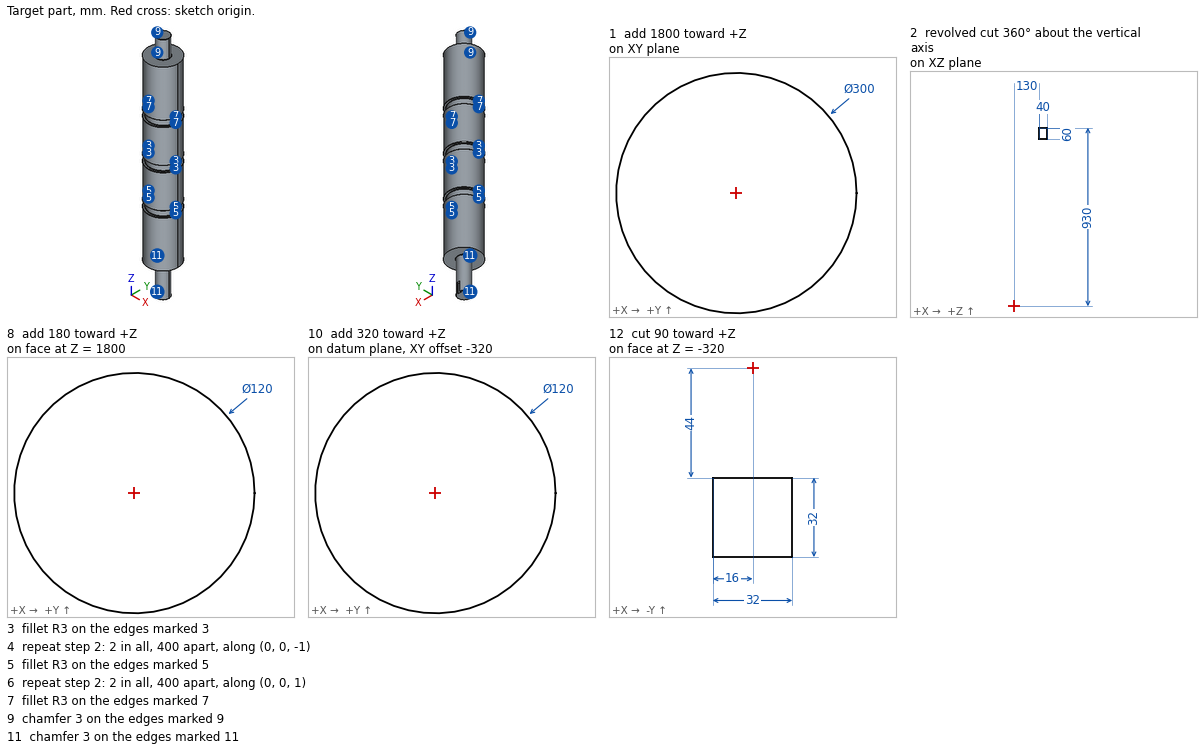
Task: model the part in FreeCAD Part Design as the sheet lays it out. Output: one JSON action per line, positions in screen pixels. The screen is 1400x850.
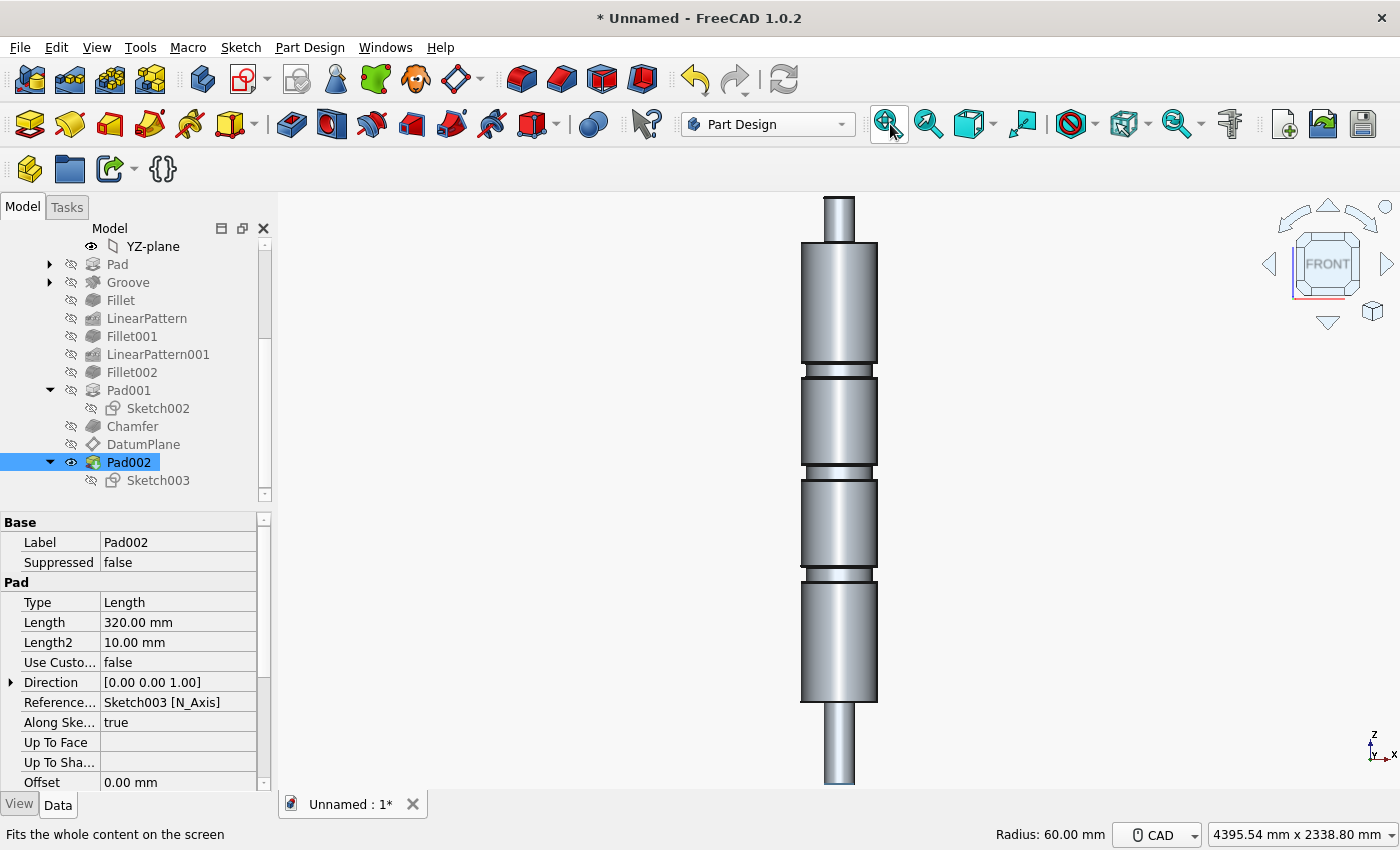
{"action": "key", "text": "3"}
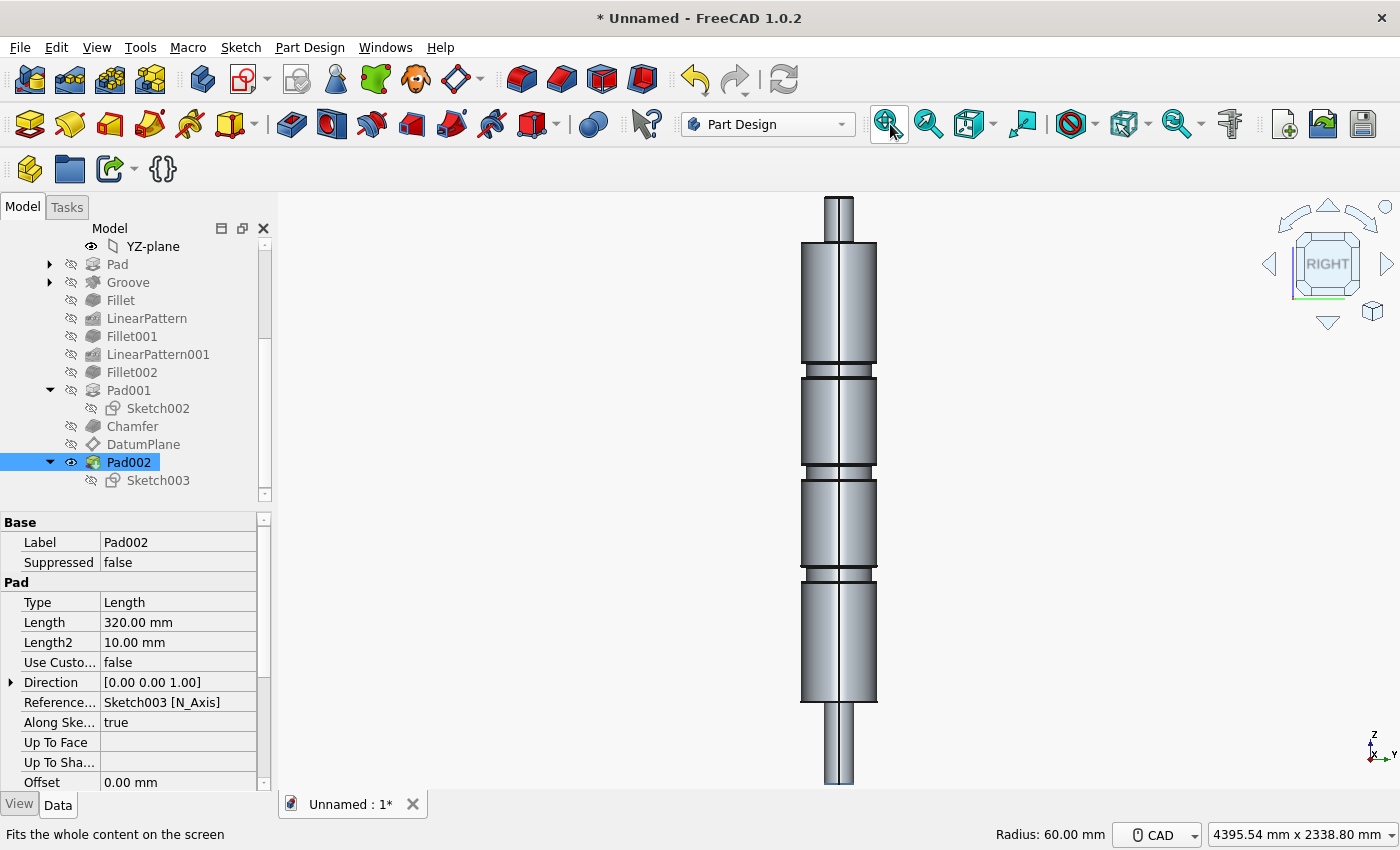
{"action": "key", "text": "5"}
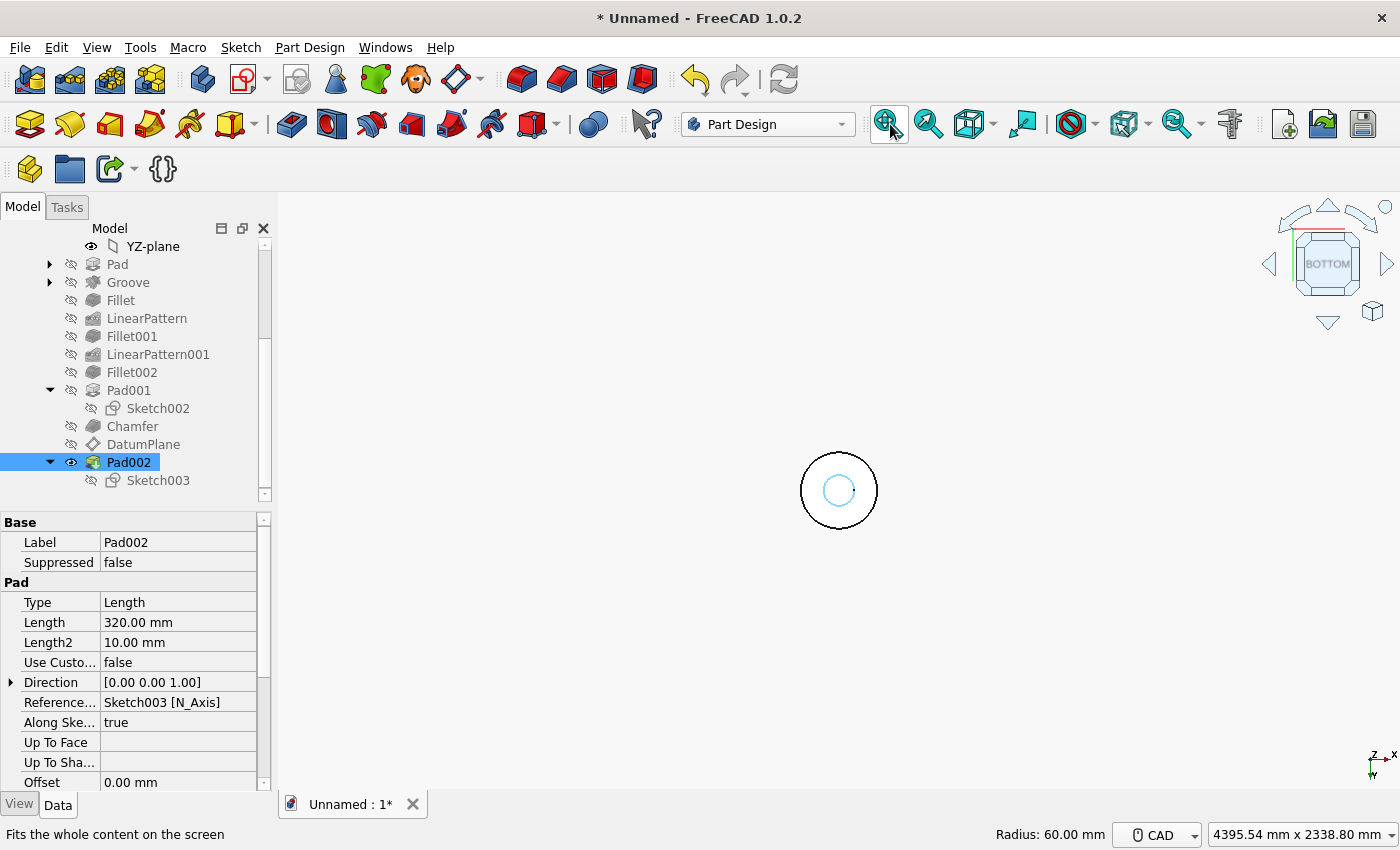
{"action": "left_click", "coordinate": [890, 124]}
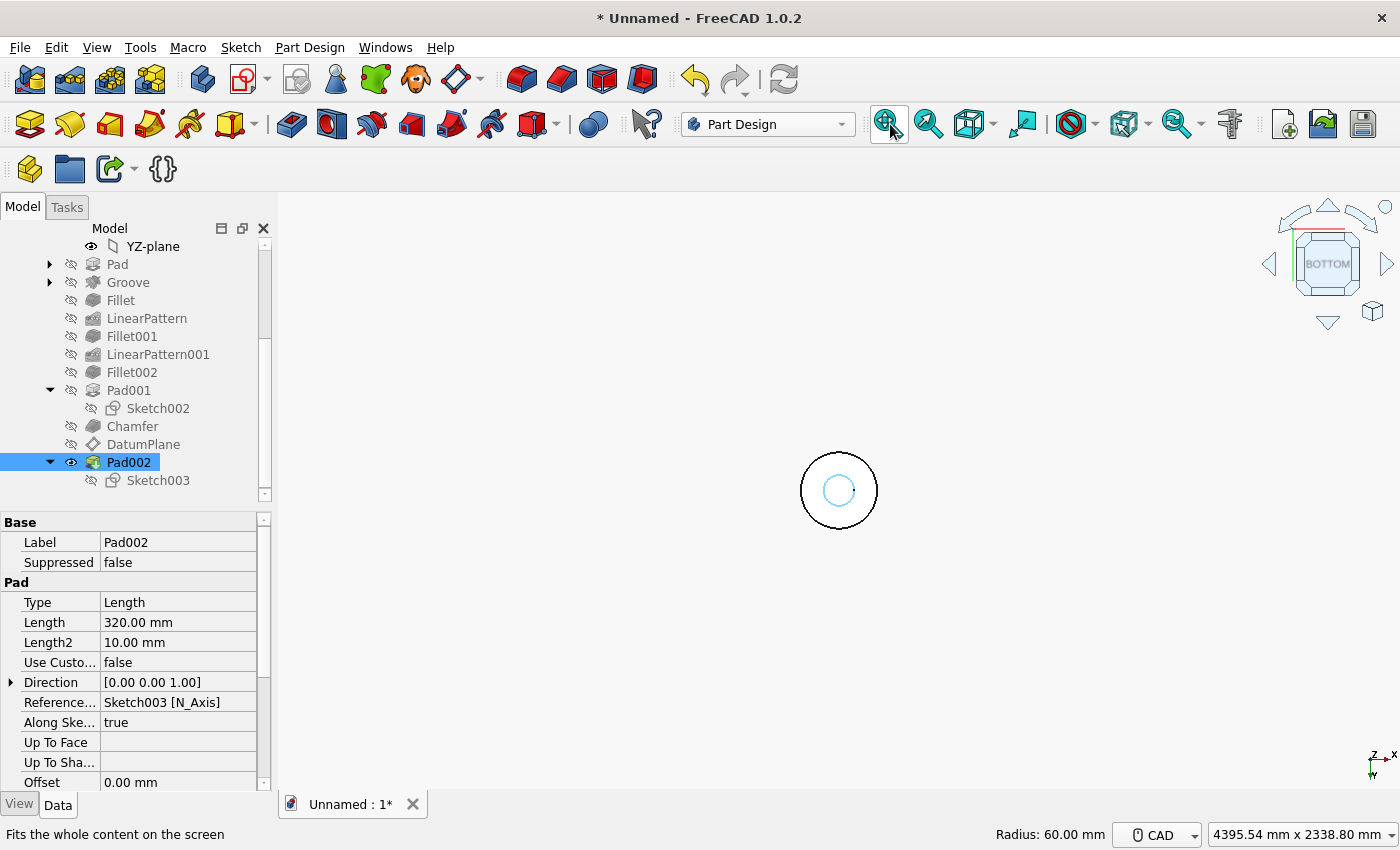
{"action": "key", "text": "4"}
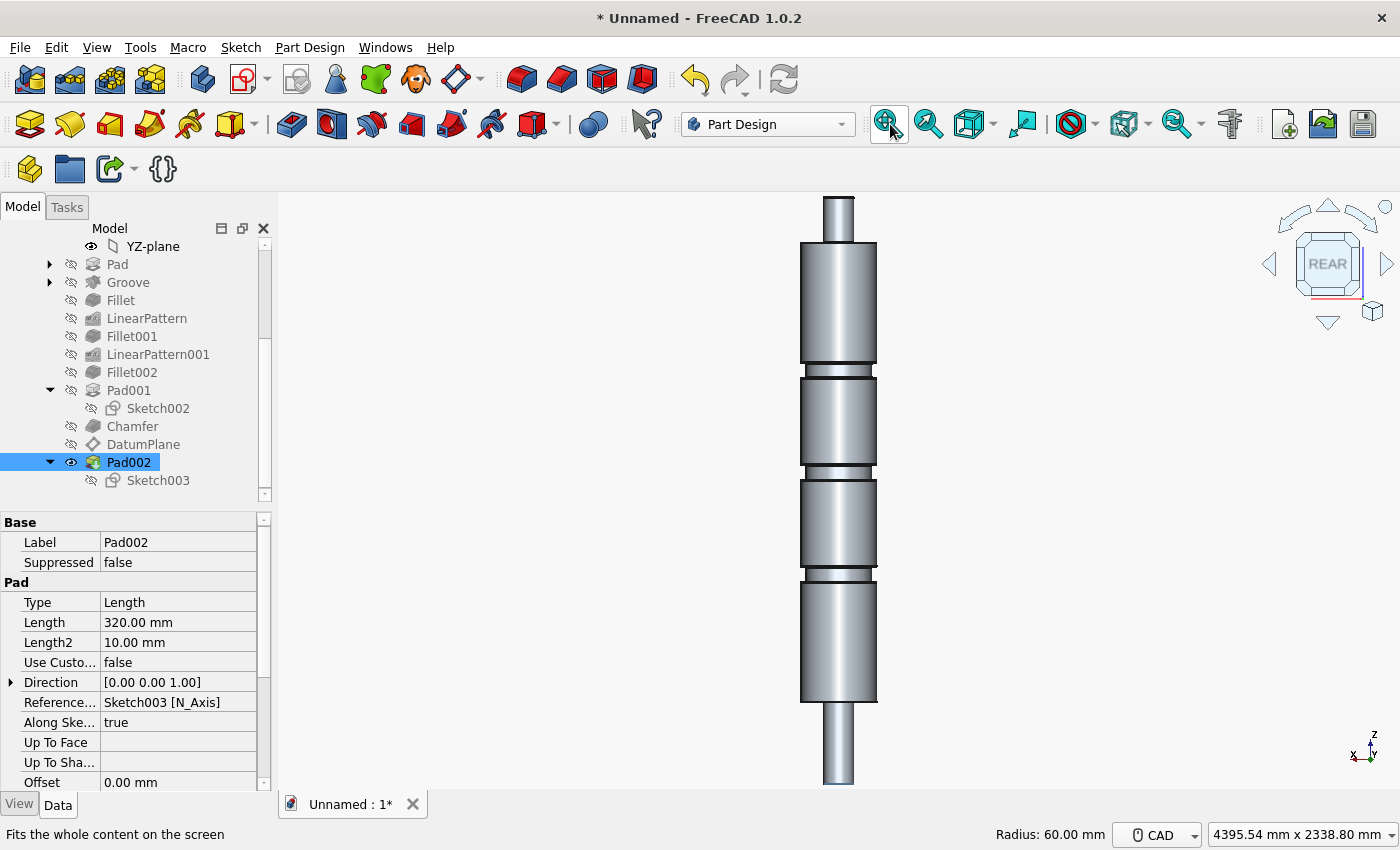
{"action": "key", "text": "6"}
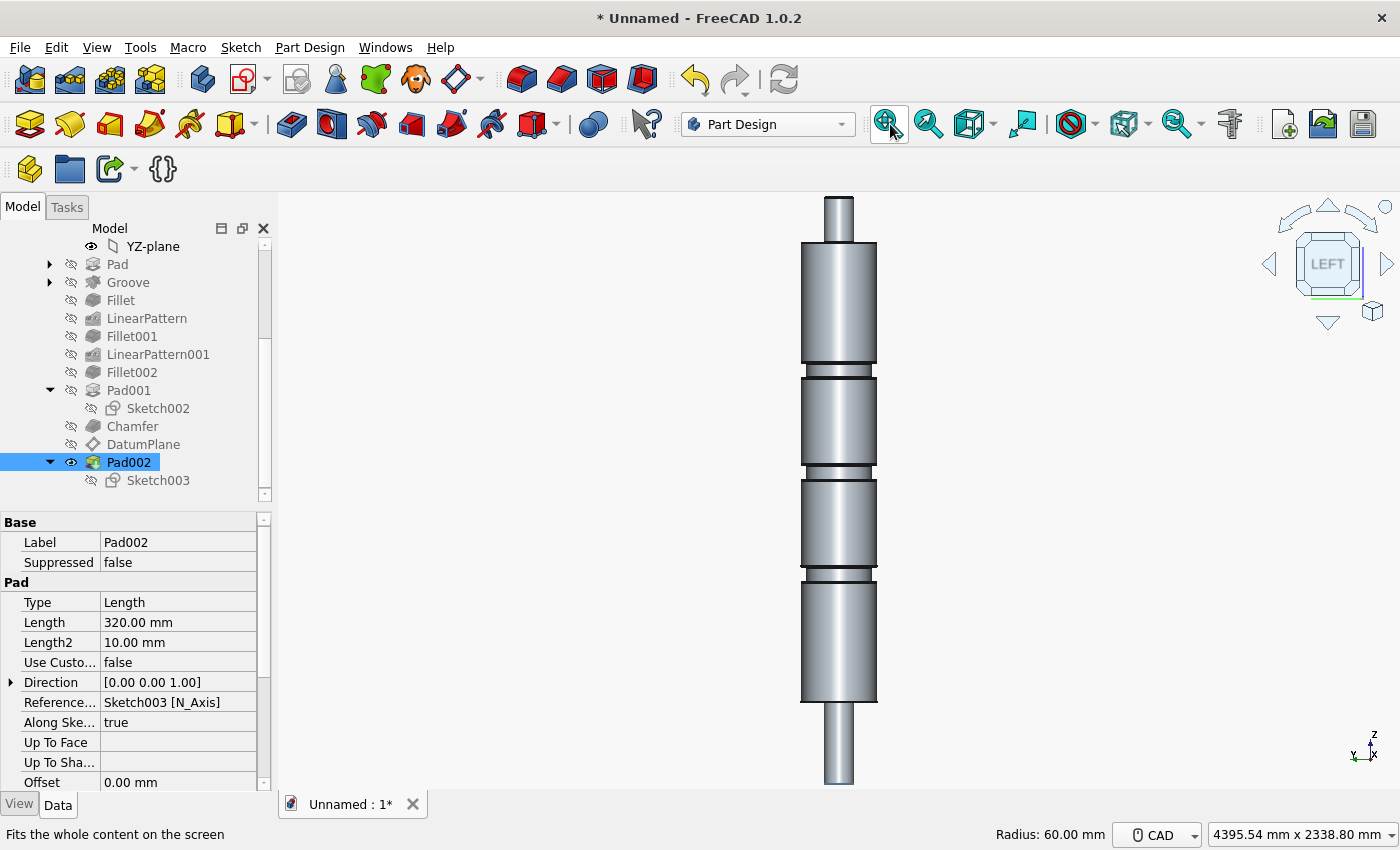
{"action": "key", "text": "v 3"}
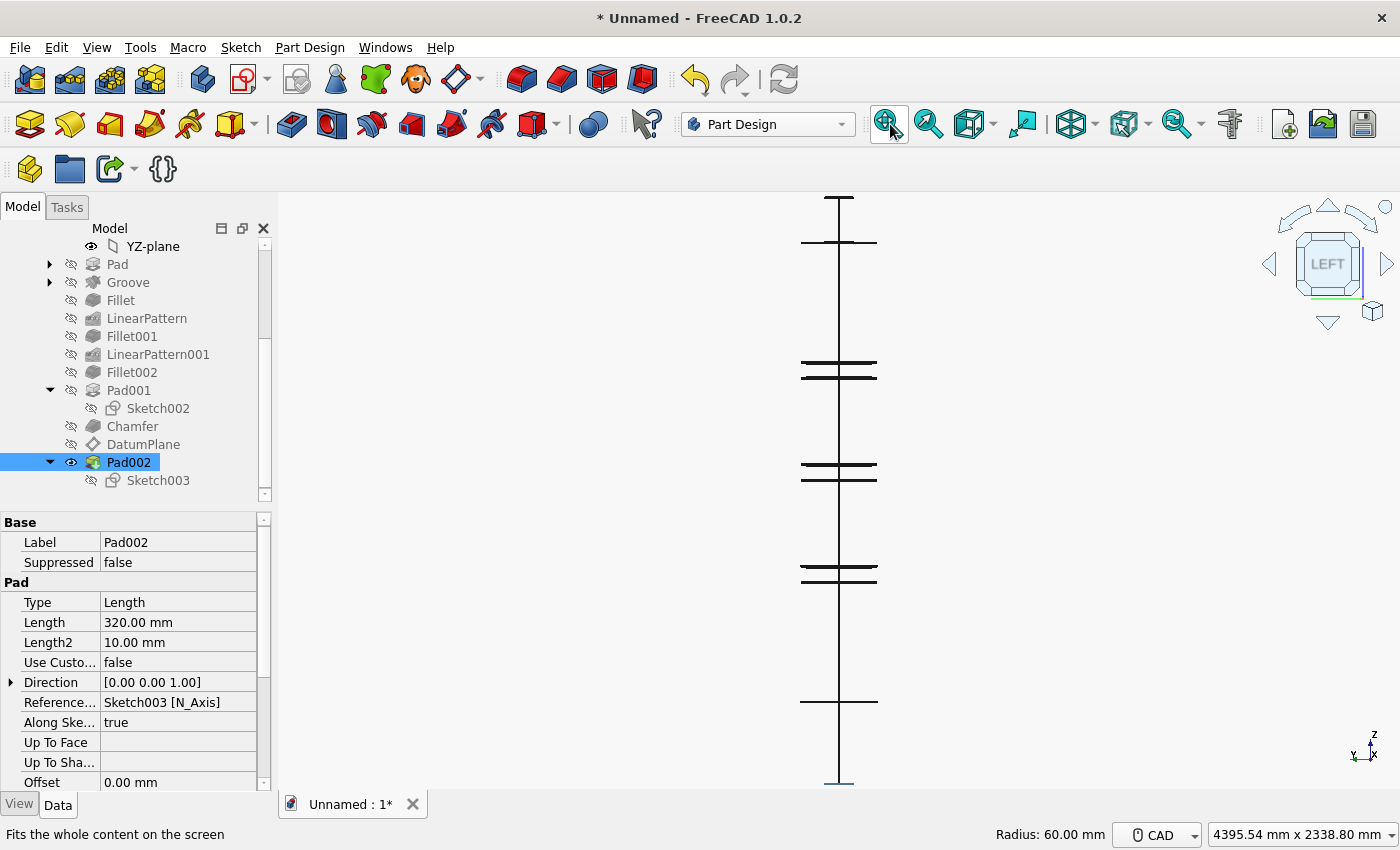
{"action": "key", "text": "0"}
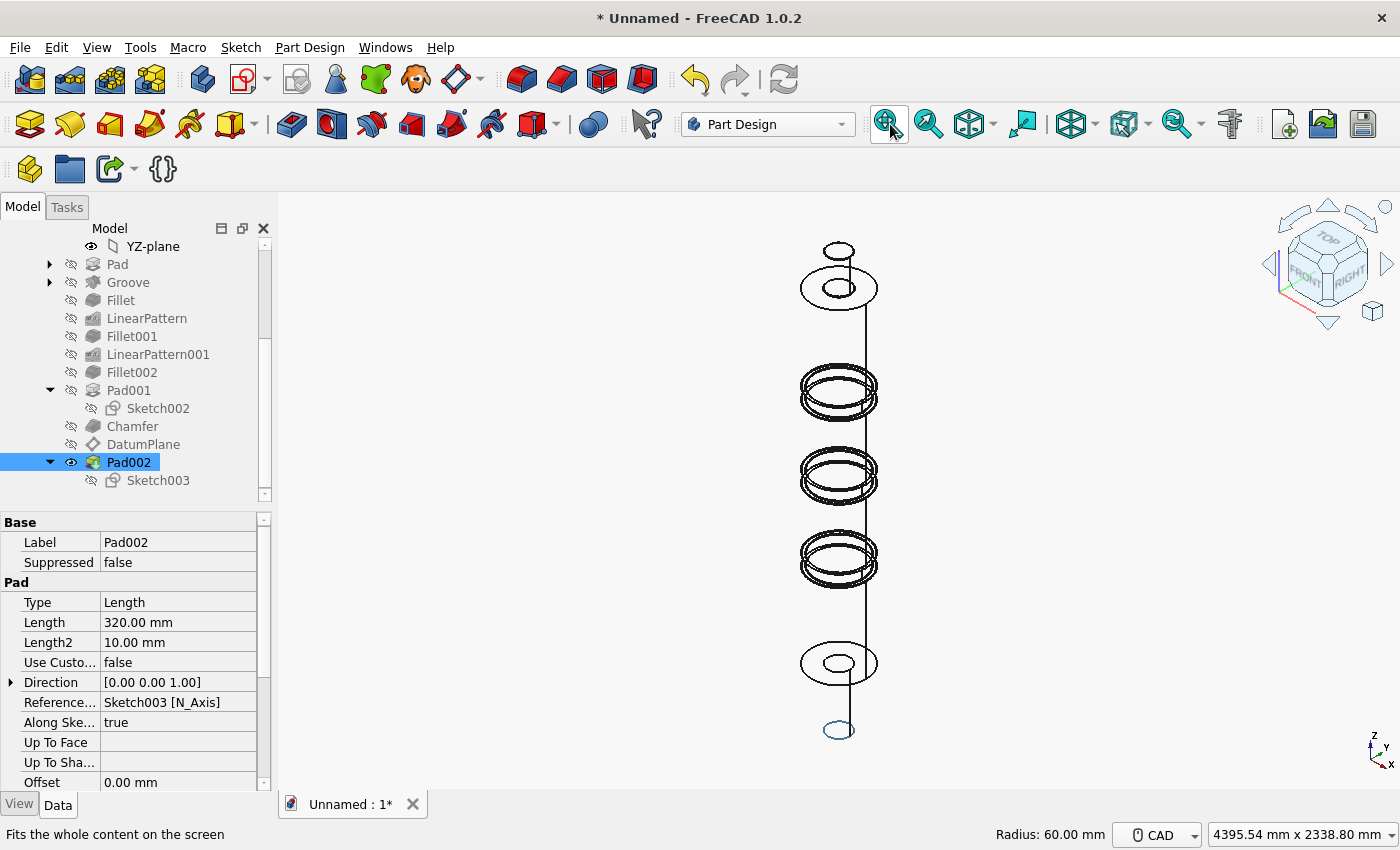
{"action": "left_click", "coordinate": [828, 656], "text": "ctrl"}